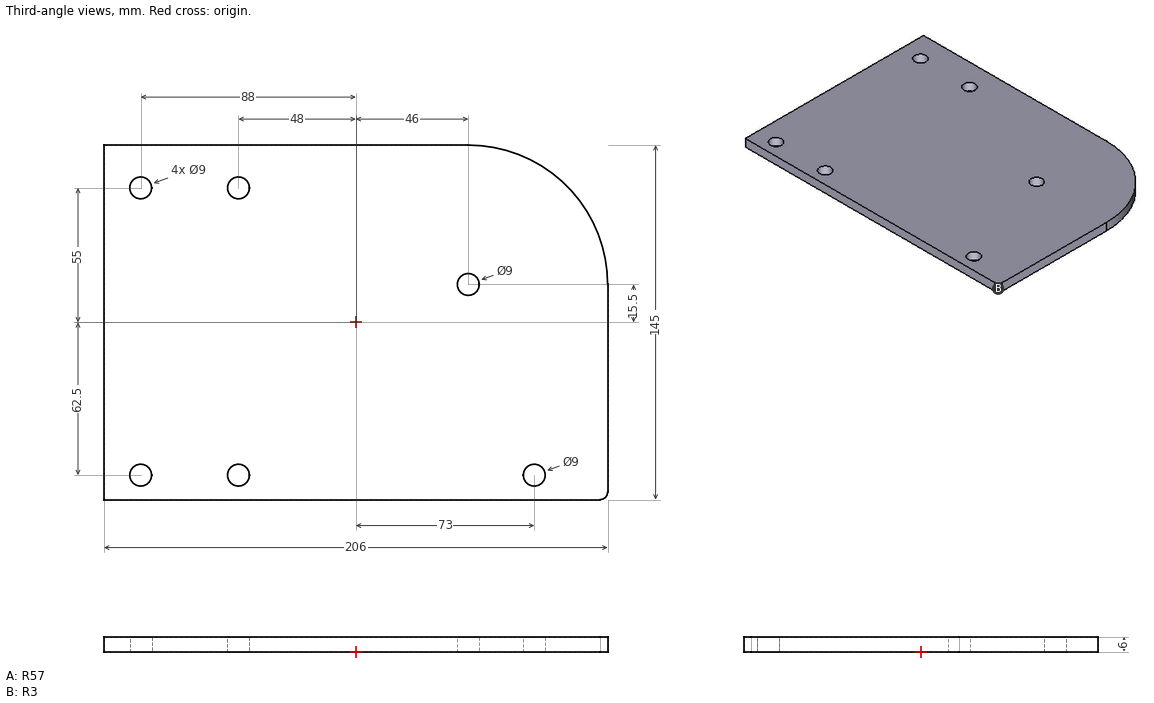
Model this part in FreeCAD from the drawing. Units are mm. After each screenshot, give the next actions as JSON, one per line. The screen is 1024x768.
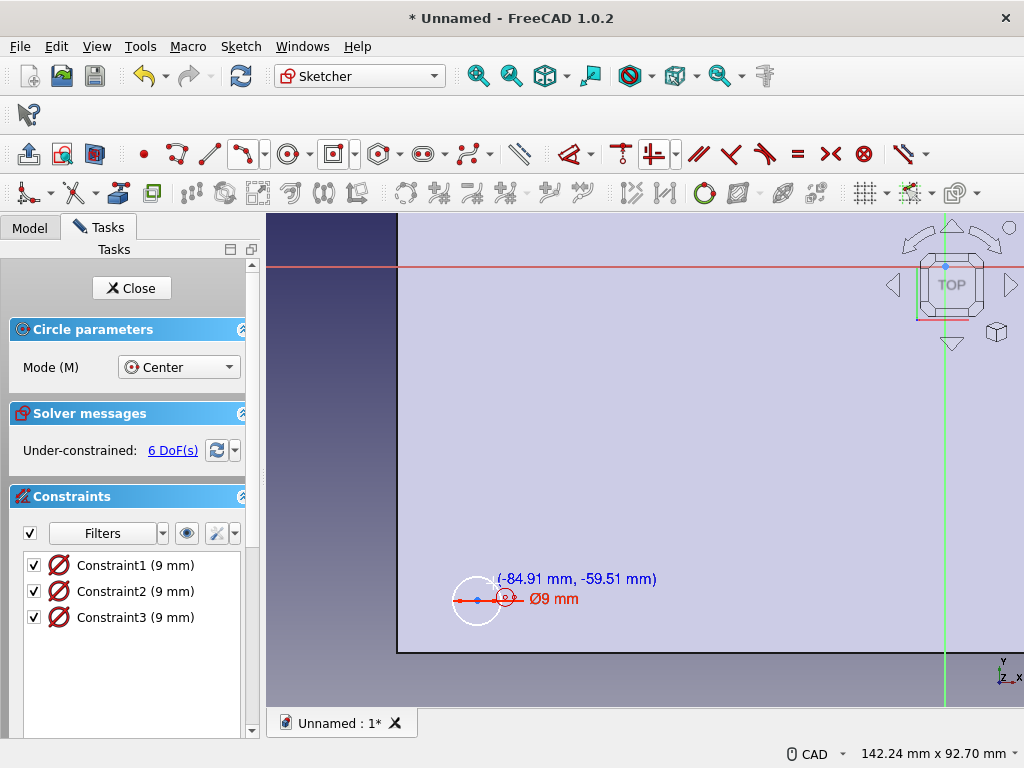
{"action": "left_click", "coordinate": [690, 600]}
{"action": "mouse_move", "coordinate": [707, 583]}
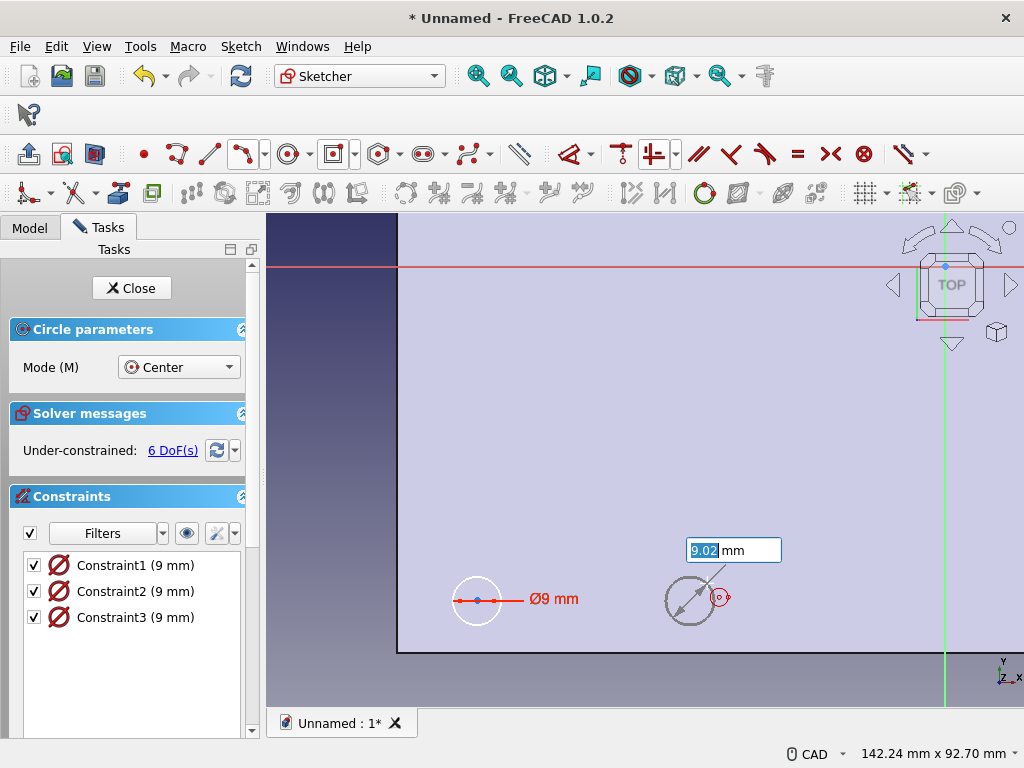
{"action": "type", "text": "9"}
{"action": "key", "text": "Return"}
{"action": "key", "text": "Escape"}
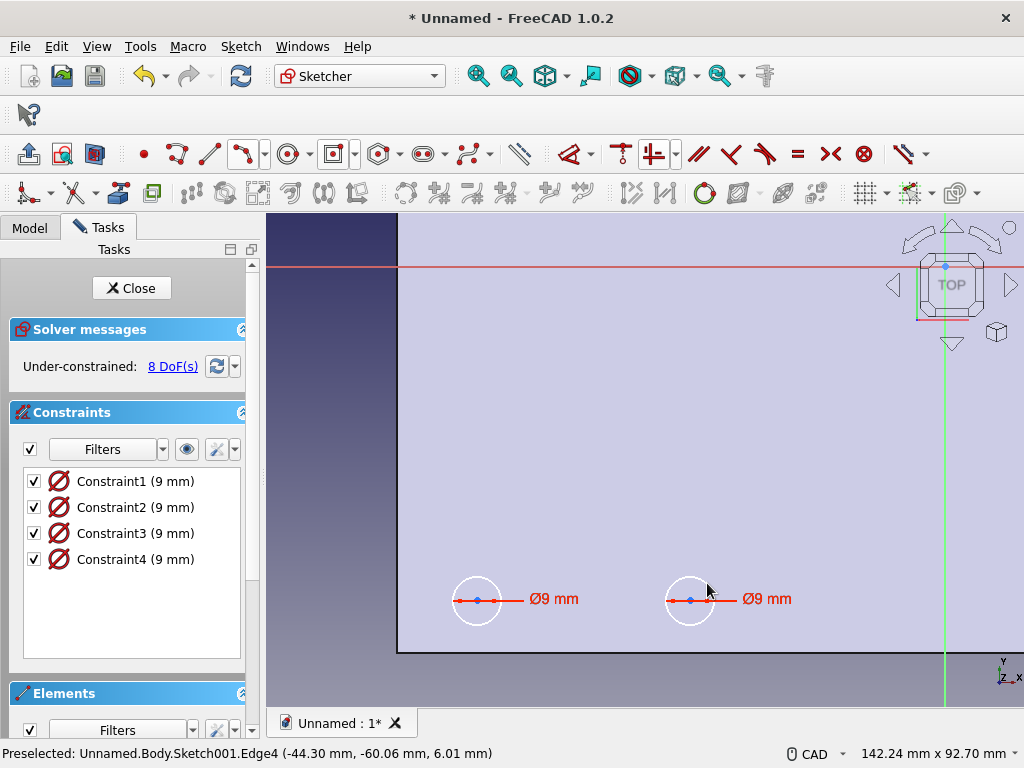
{"action": "scroll", "coordinate": [477, 601], "scroll_direction": "down", "scroll_amount": 4}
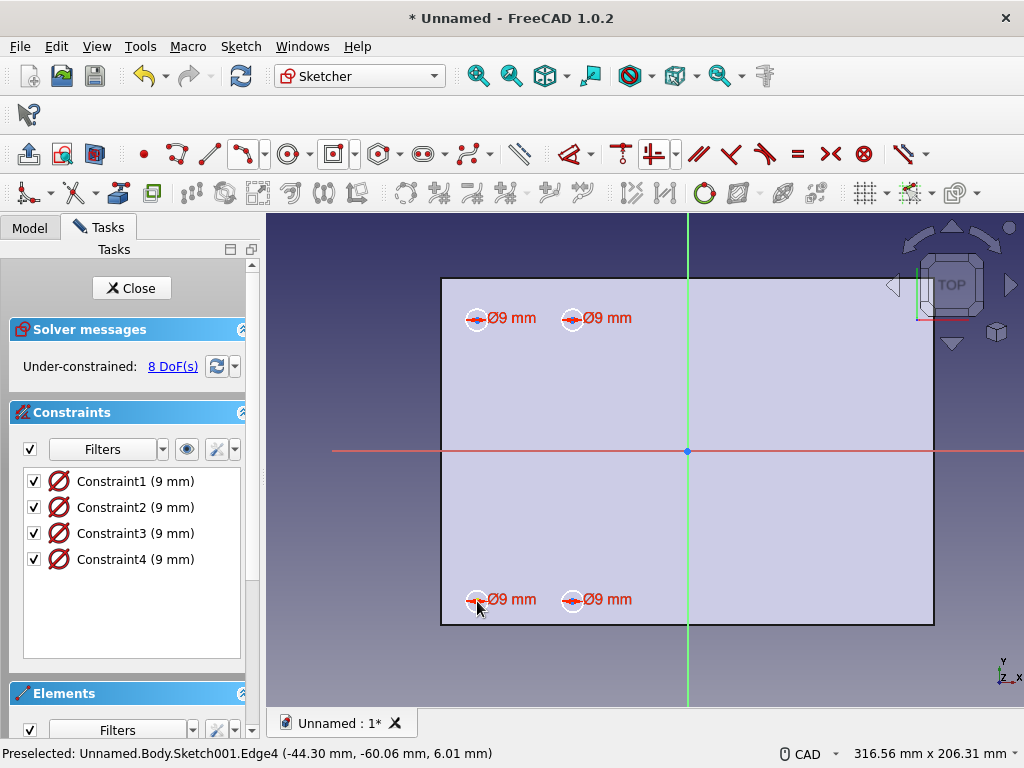
{"action": "left_click", "coordinate": [477, 320]}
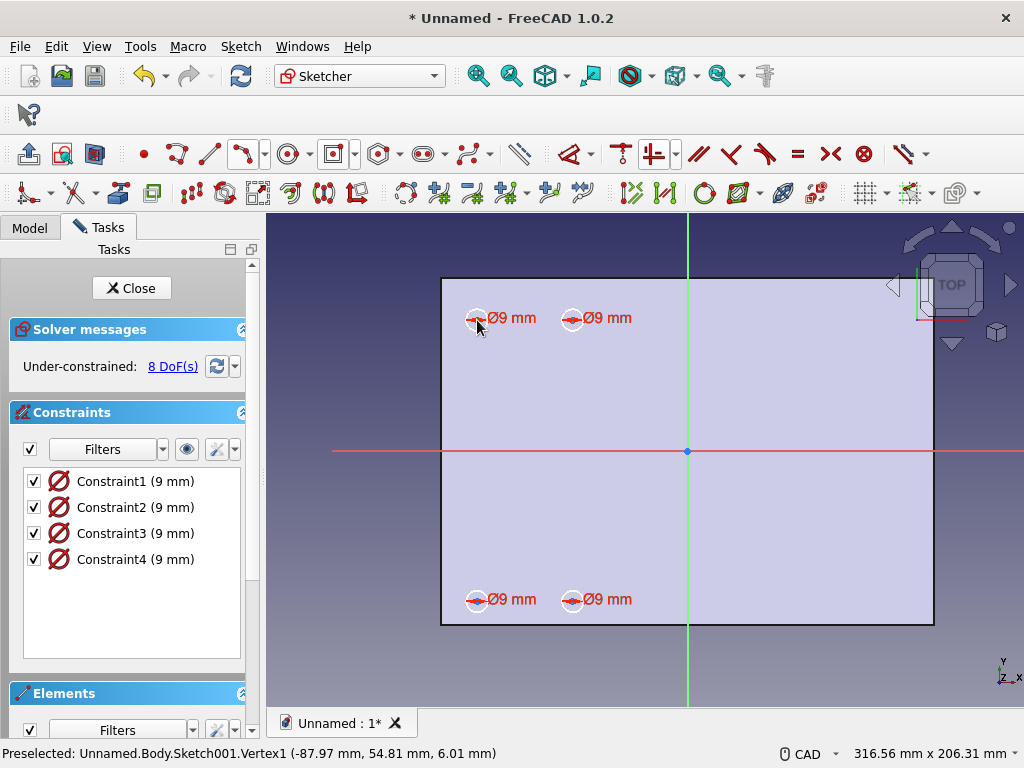
{"action": "left_click", "coordinate": [573, 320]}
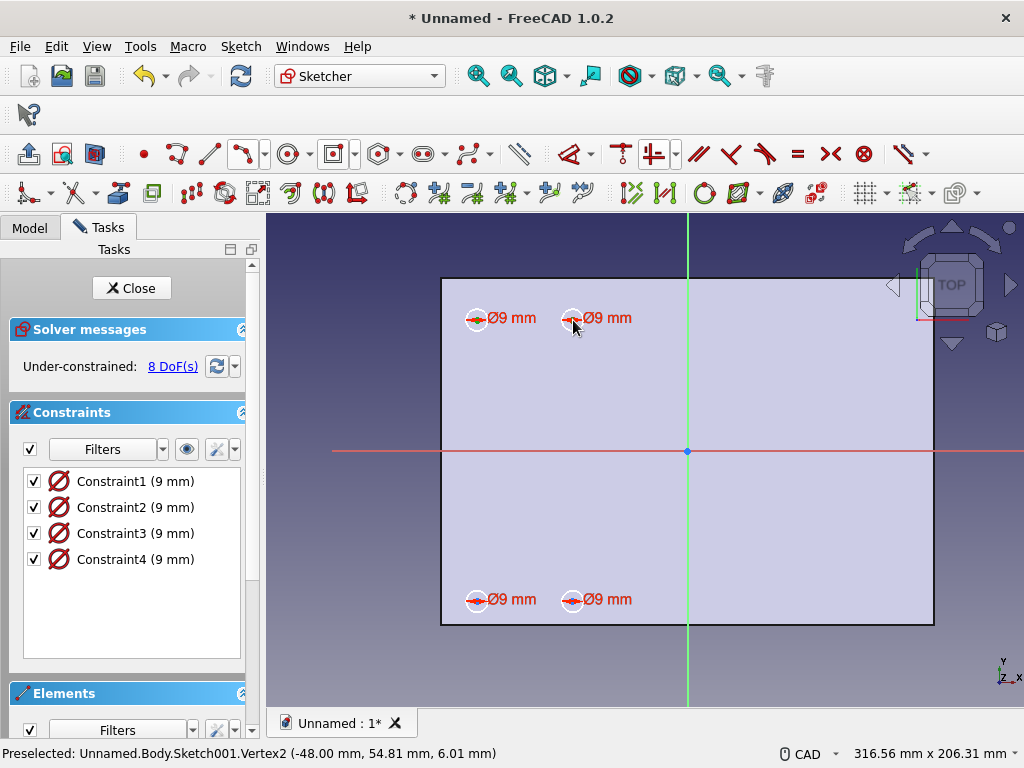
{"action": "key", "text": "h"}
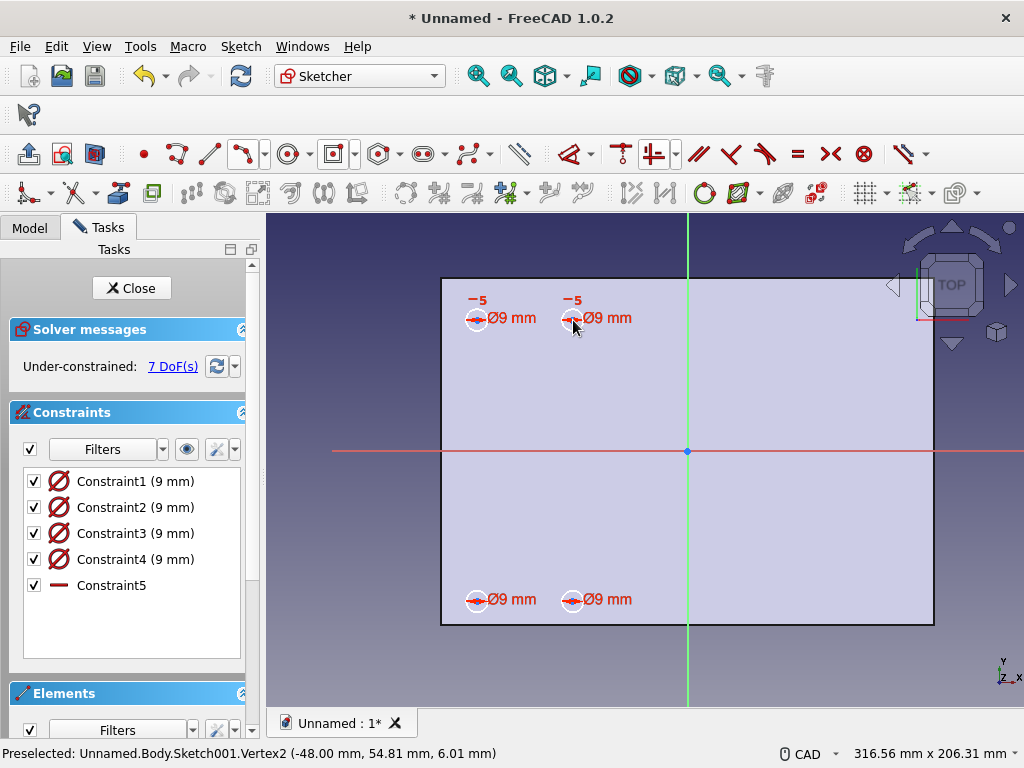
{"action": "left_click", "coordinate": [477, 320]}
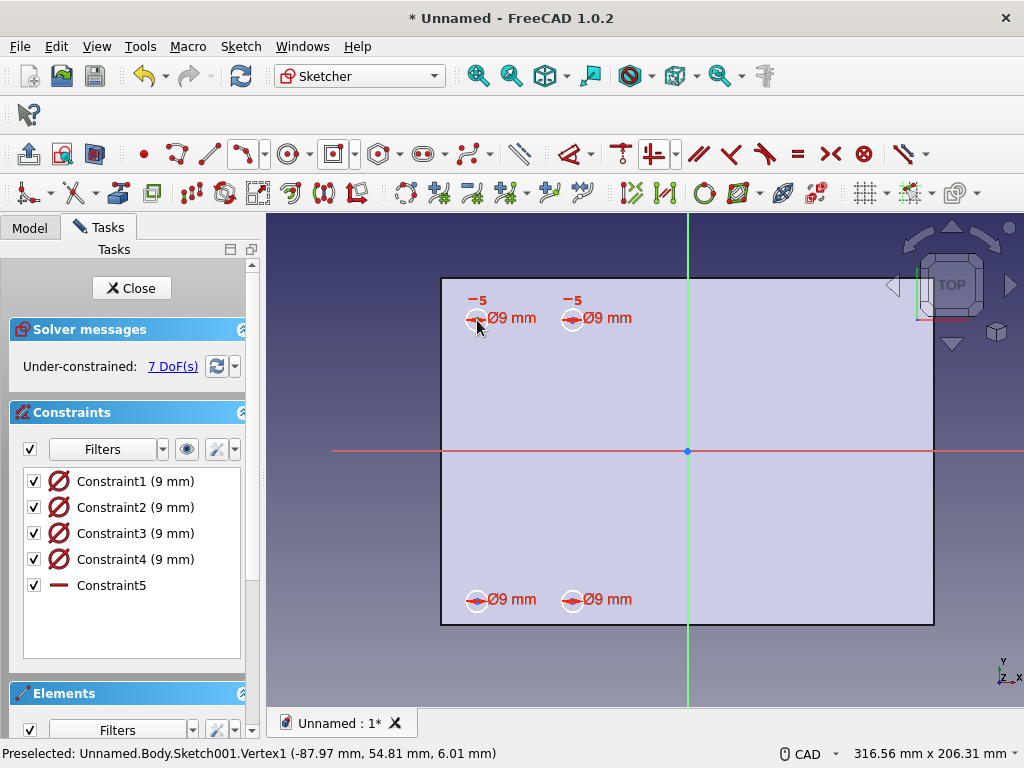
{"action": "left_click", "coordinate": [477, 601]}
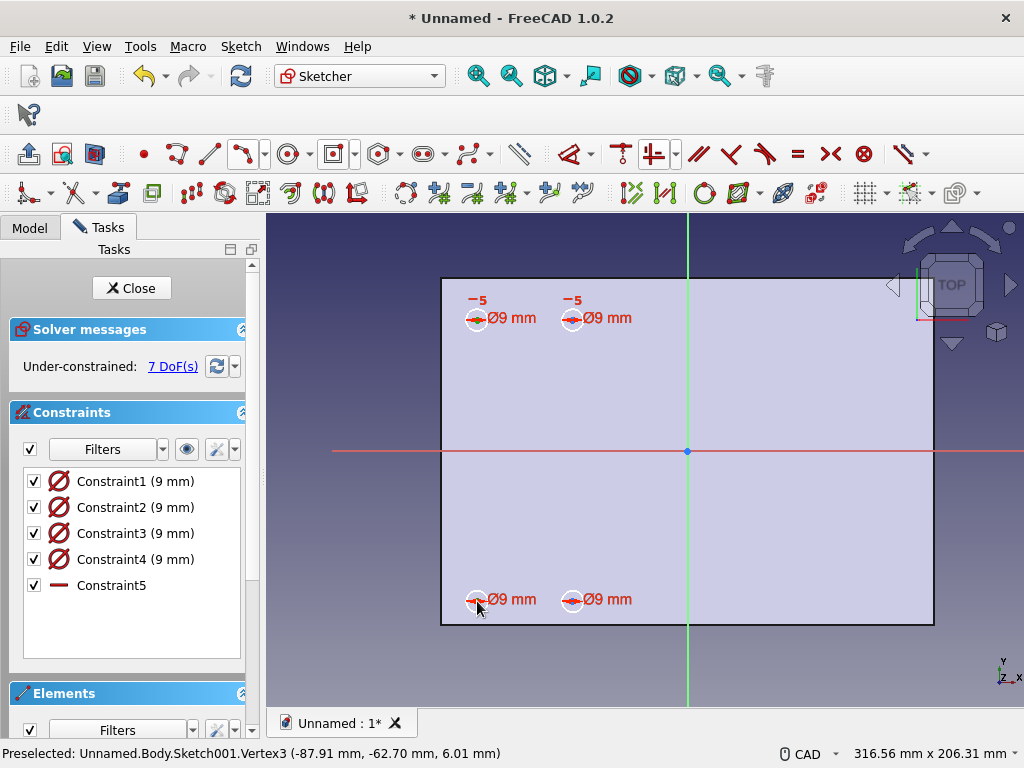
{"action": "key", "text": "v"}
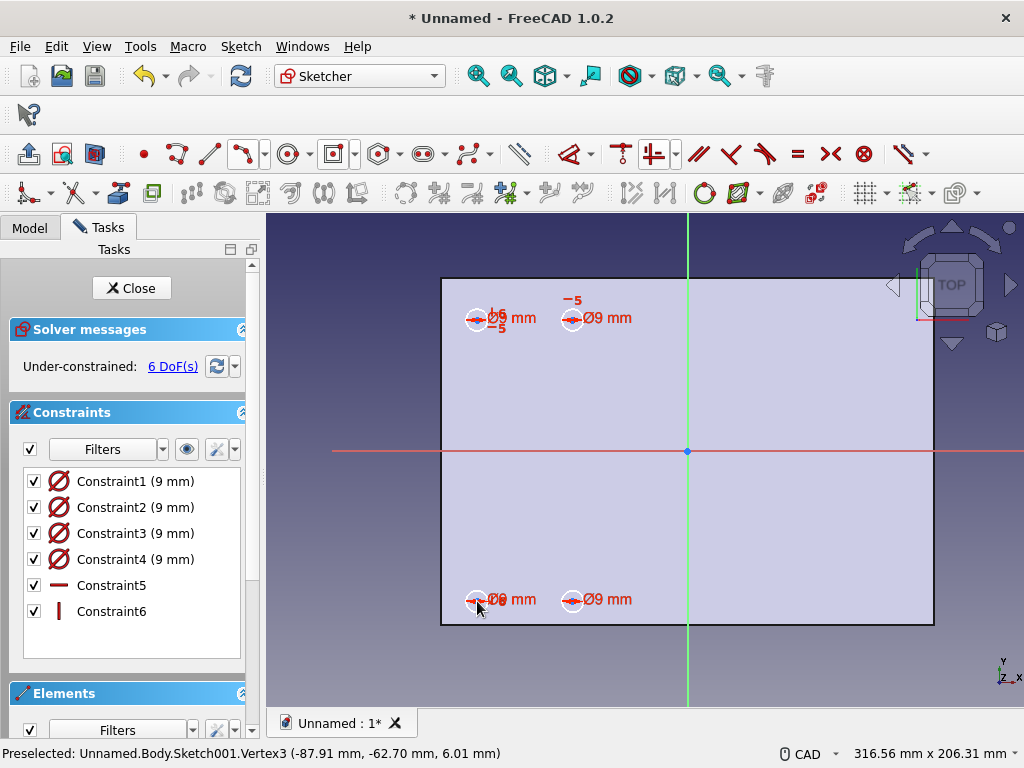
{"action": "left_click", "coordinate": [573, 320]}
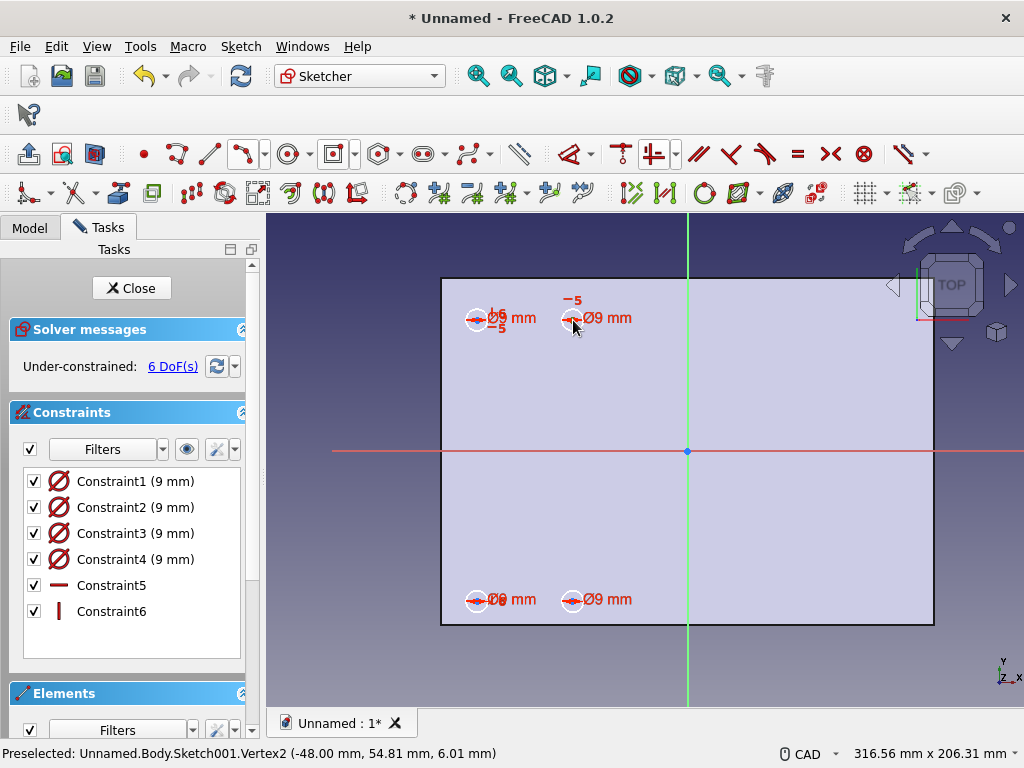
{"action": "left_click", "coordinate": [573, 601]}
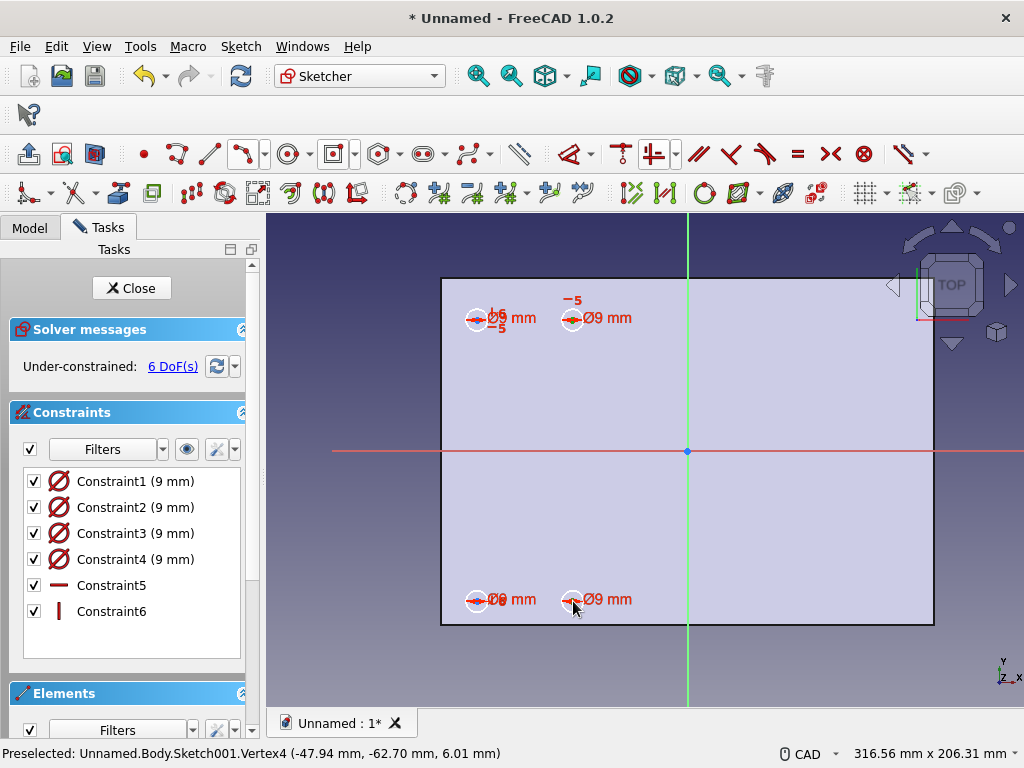
{"action": "key", "text": "v"}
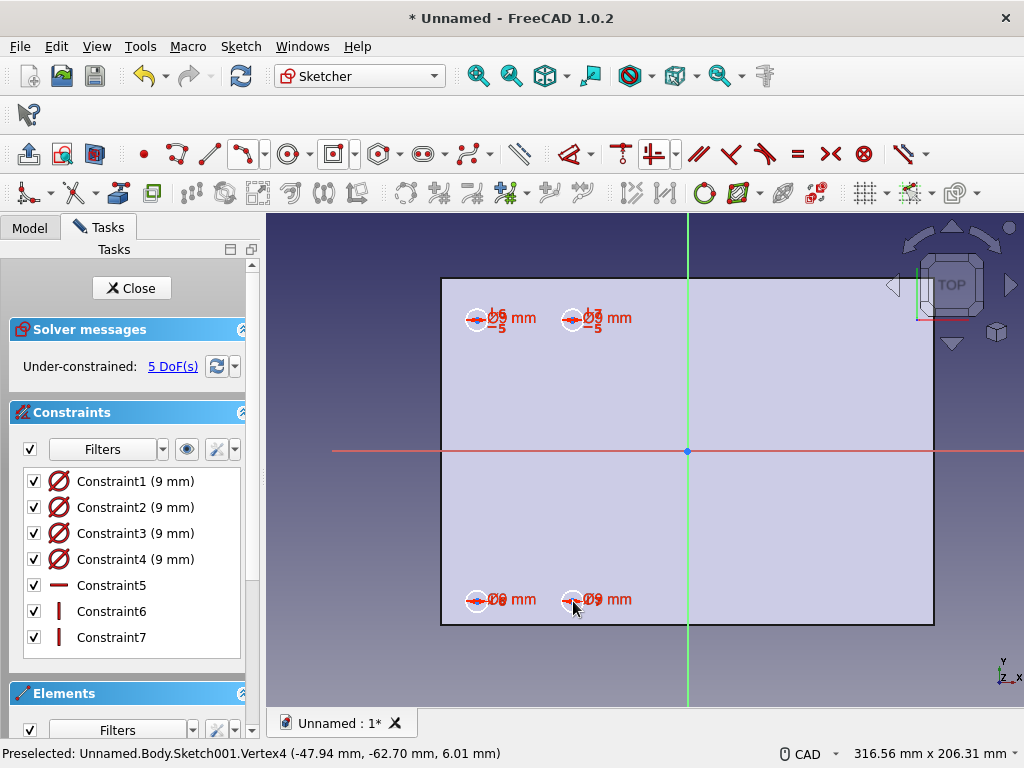
{"action": "left_click", "coordinate": [477, 601]}